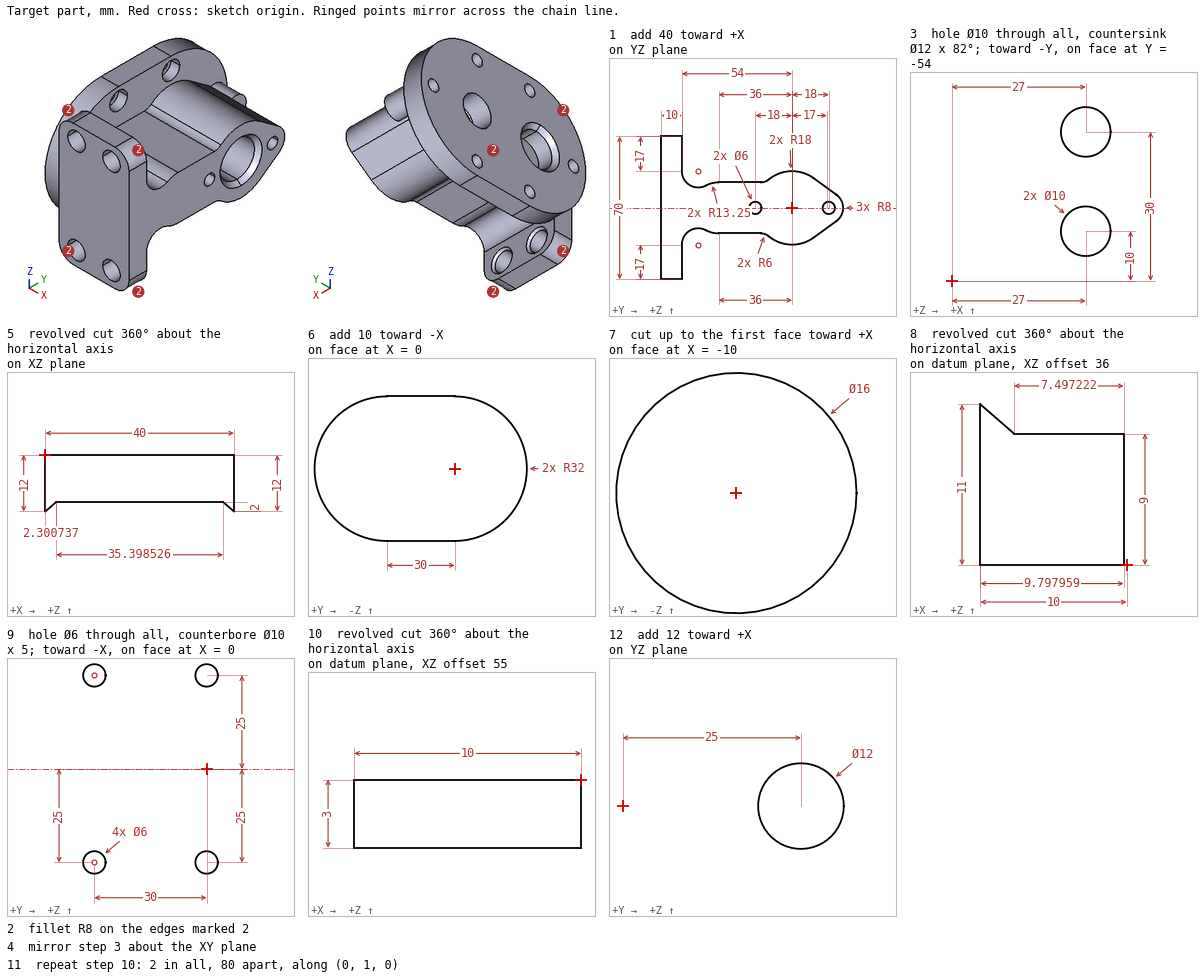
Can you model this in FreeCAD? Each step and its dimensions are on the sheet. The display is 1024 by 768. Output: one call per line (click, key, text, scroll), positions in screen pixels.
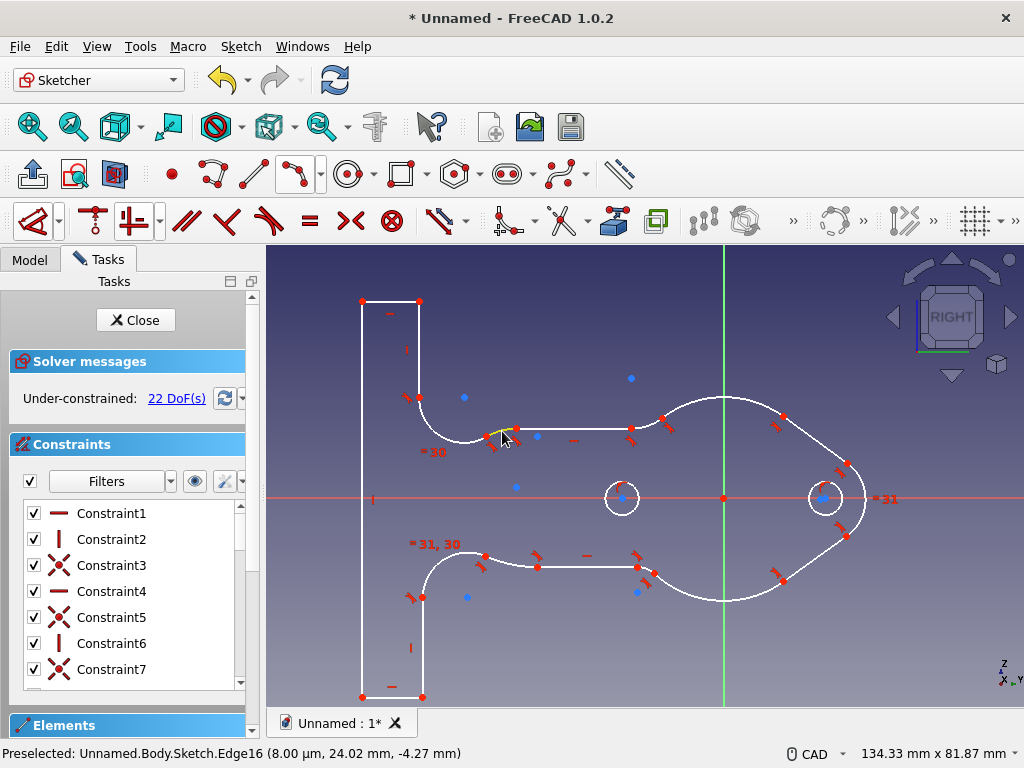
click(501, 431)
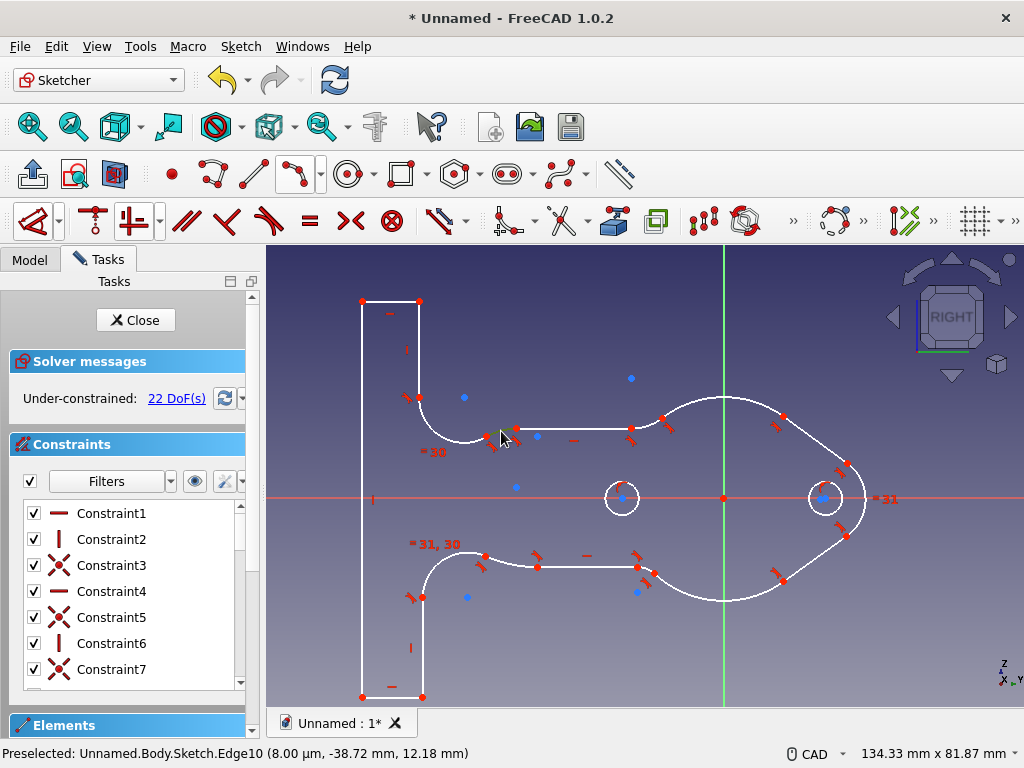
click(501, 562)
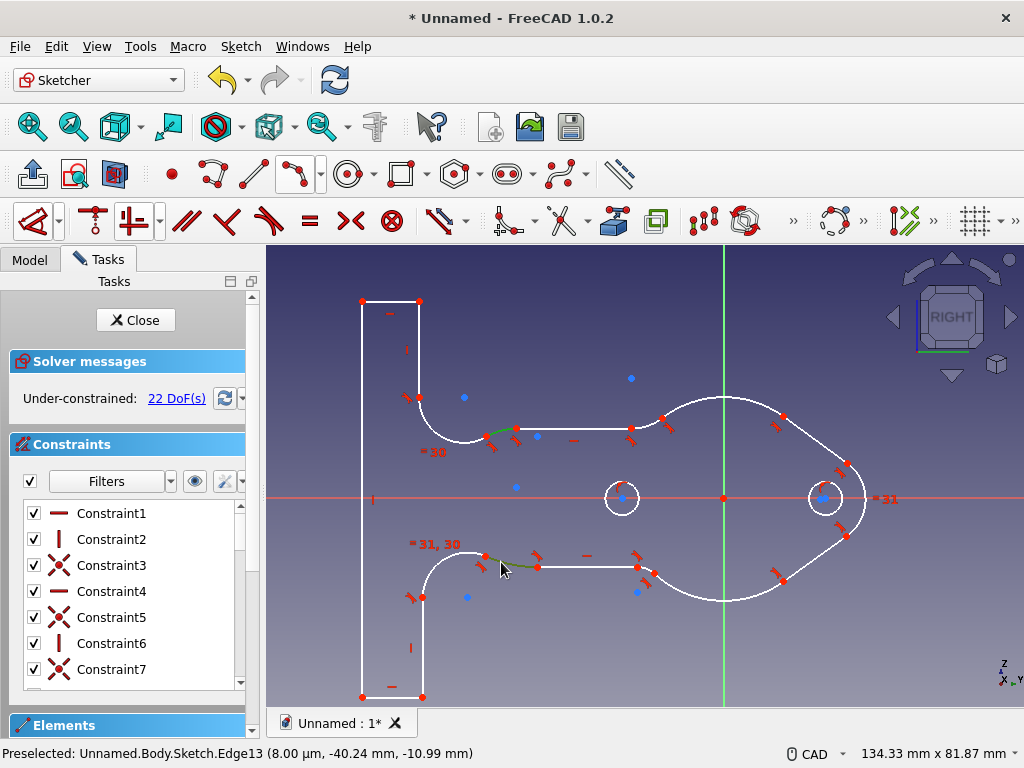
click(310, 222)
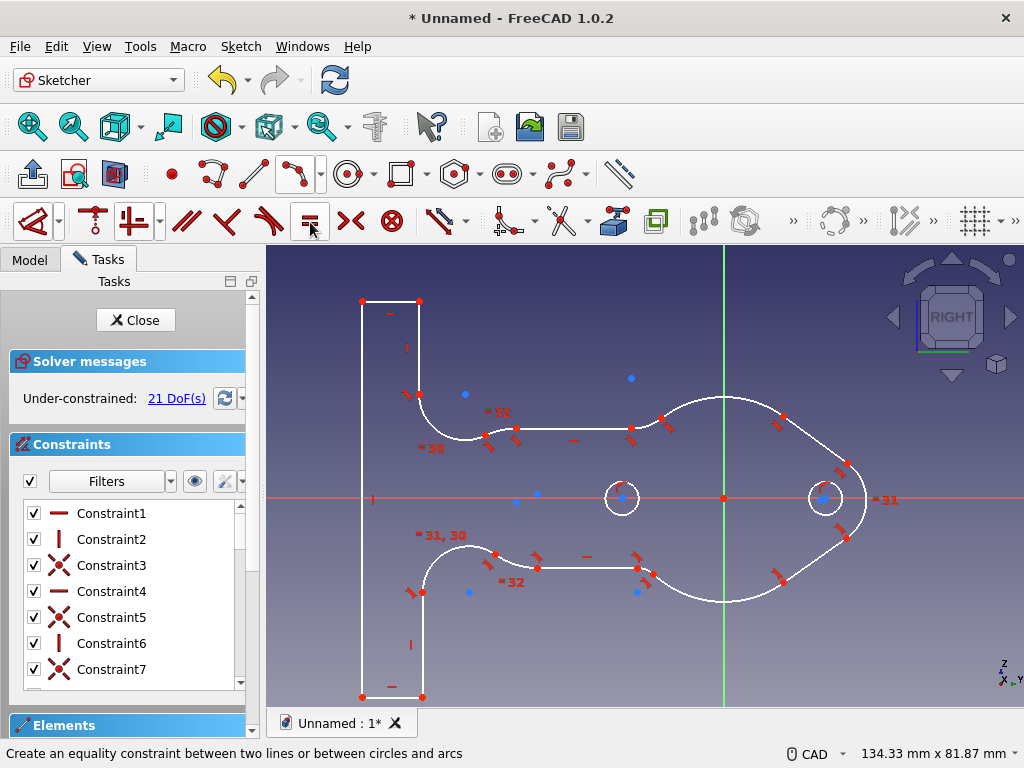
click(690, 596)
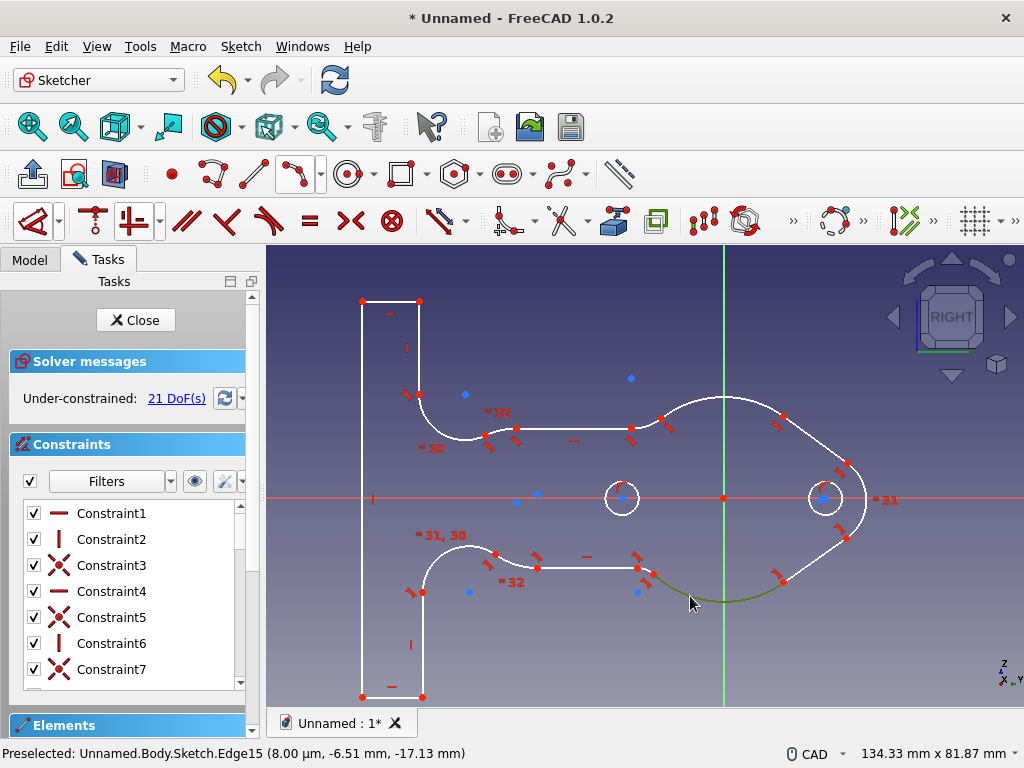
click(749, 400)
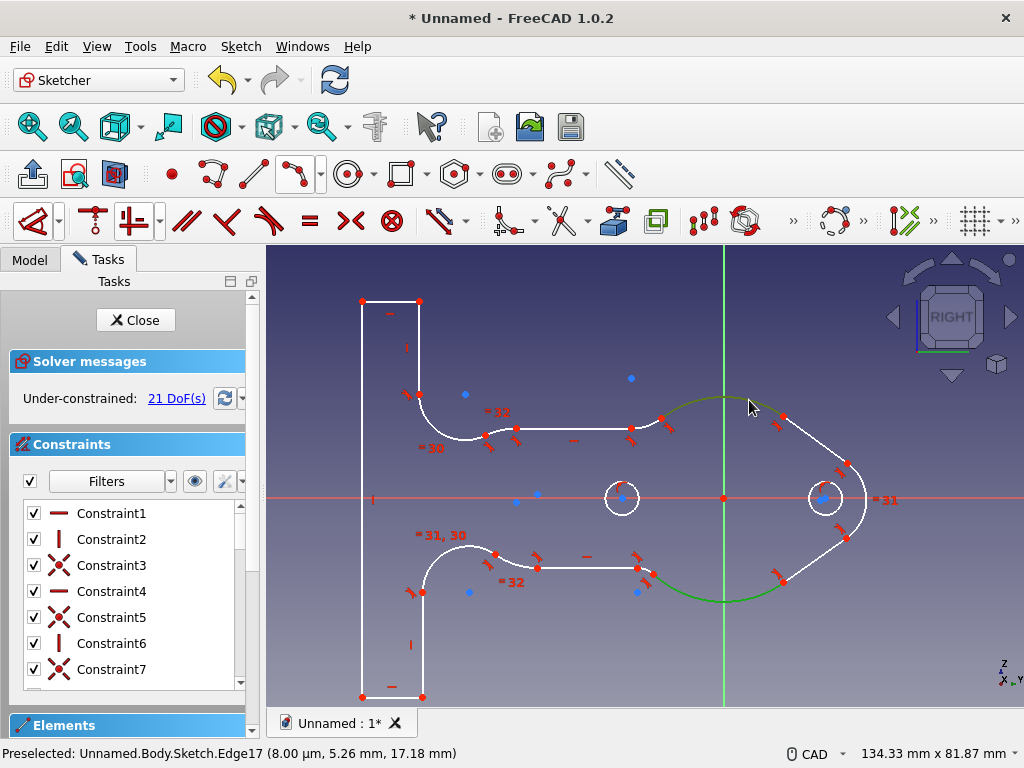
click(310, 222)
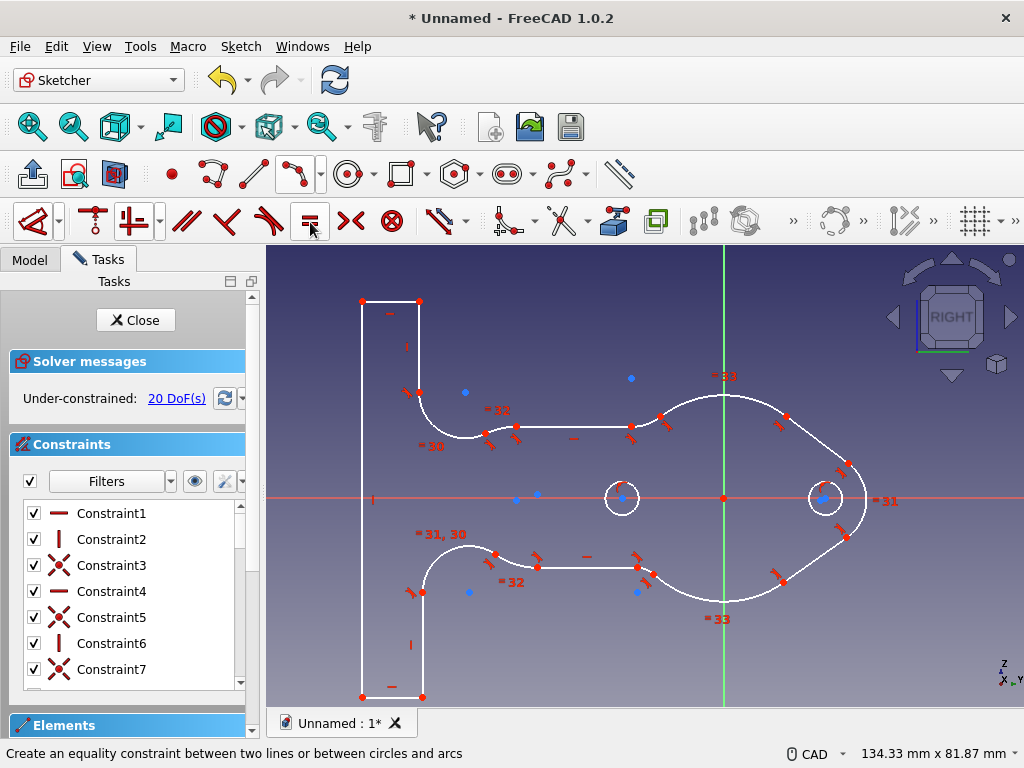
scroll(646, 570, up, 3)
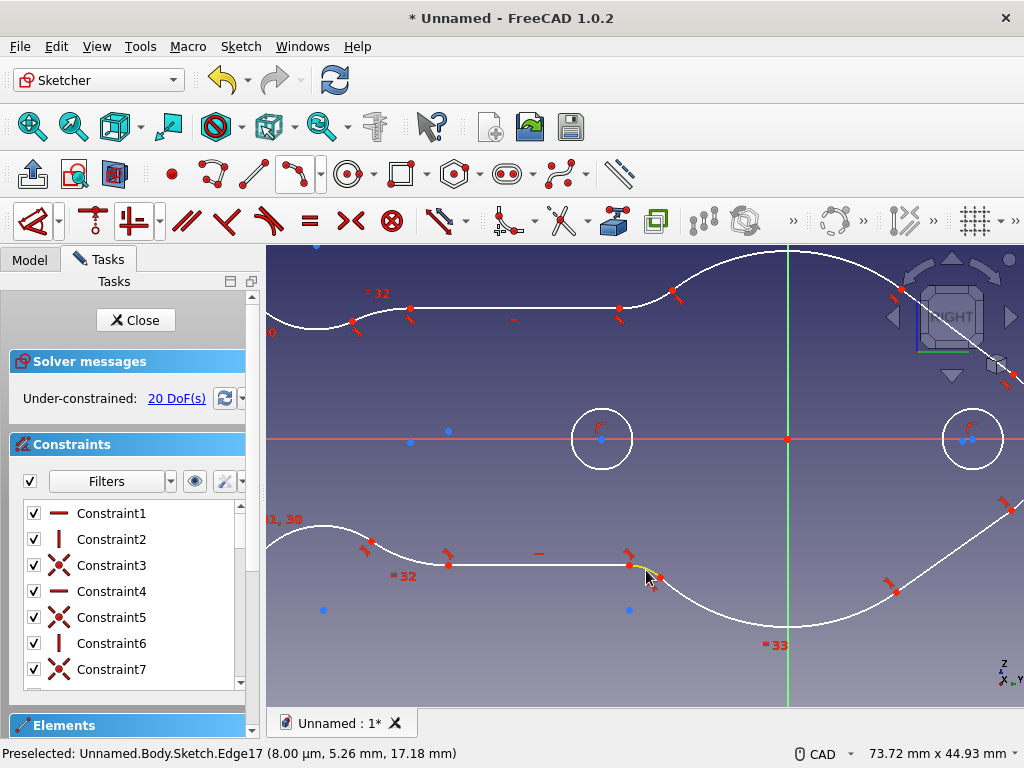
click(646, 569)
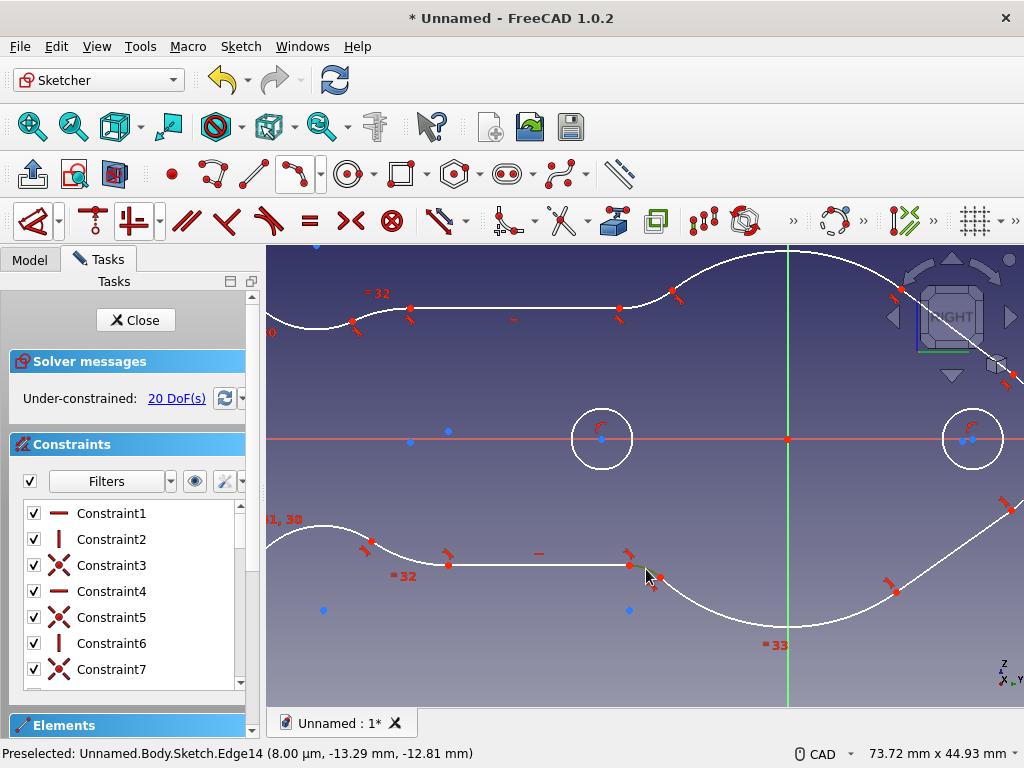
click(636, 307)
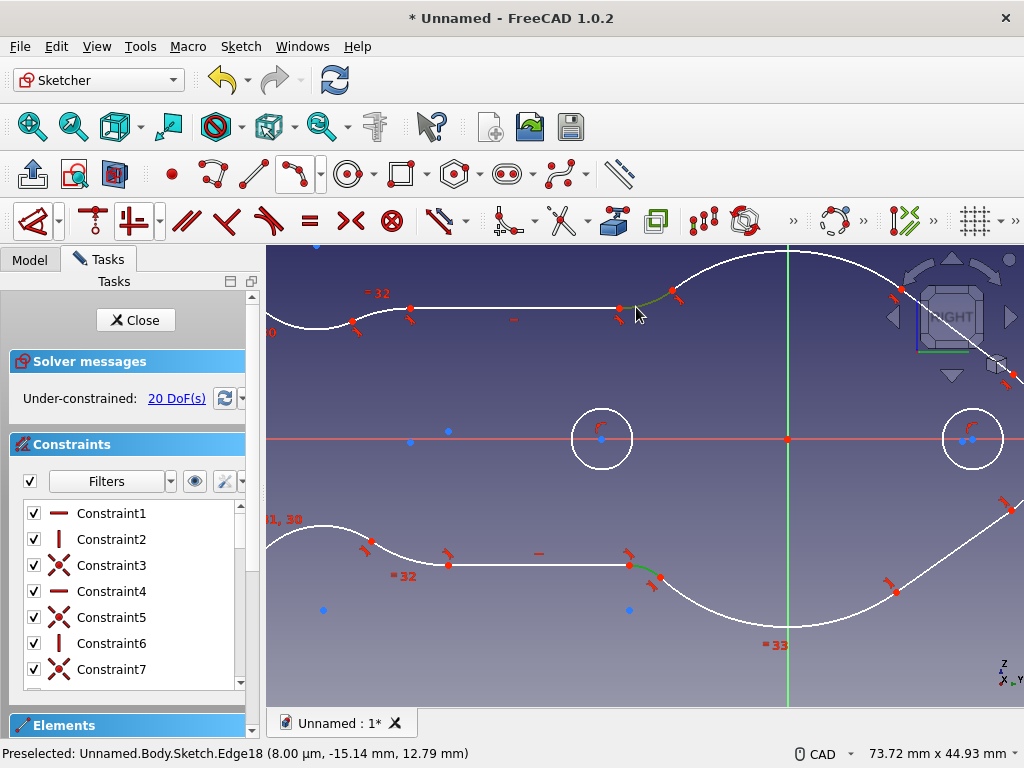
click(310, 222)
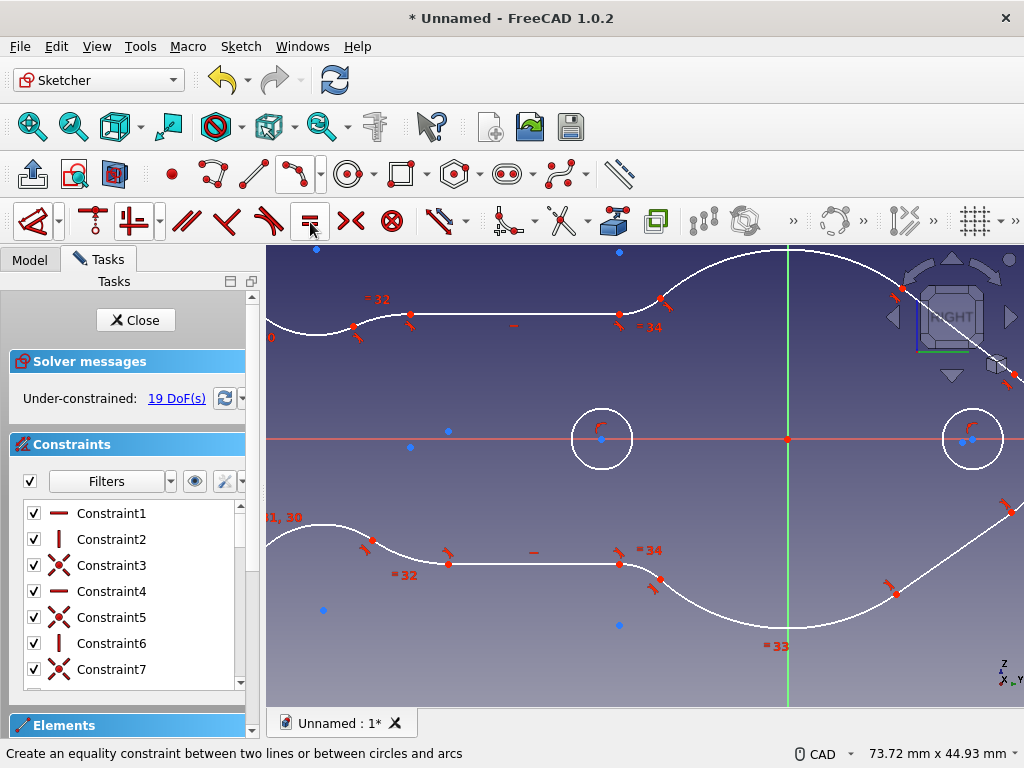
click(623, 418)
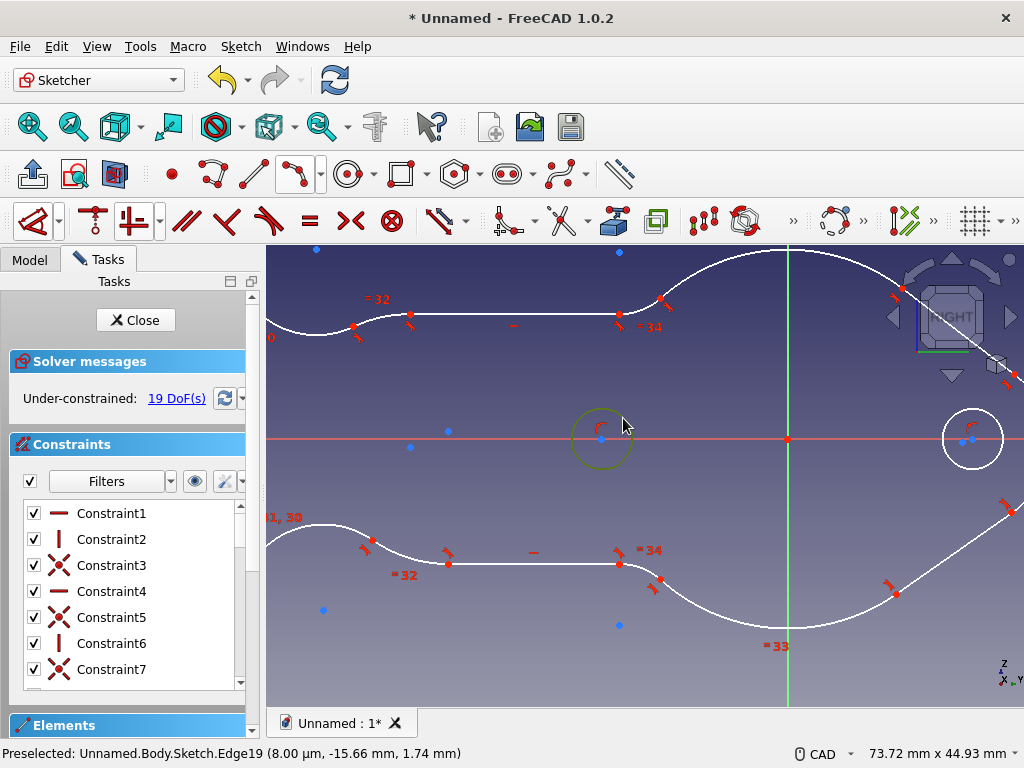
scroll(570, 497, down, 5)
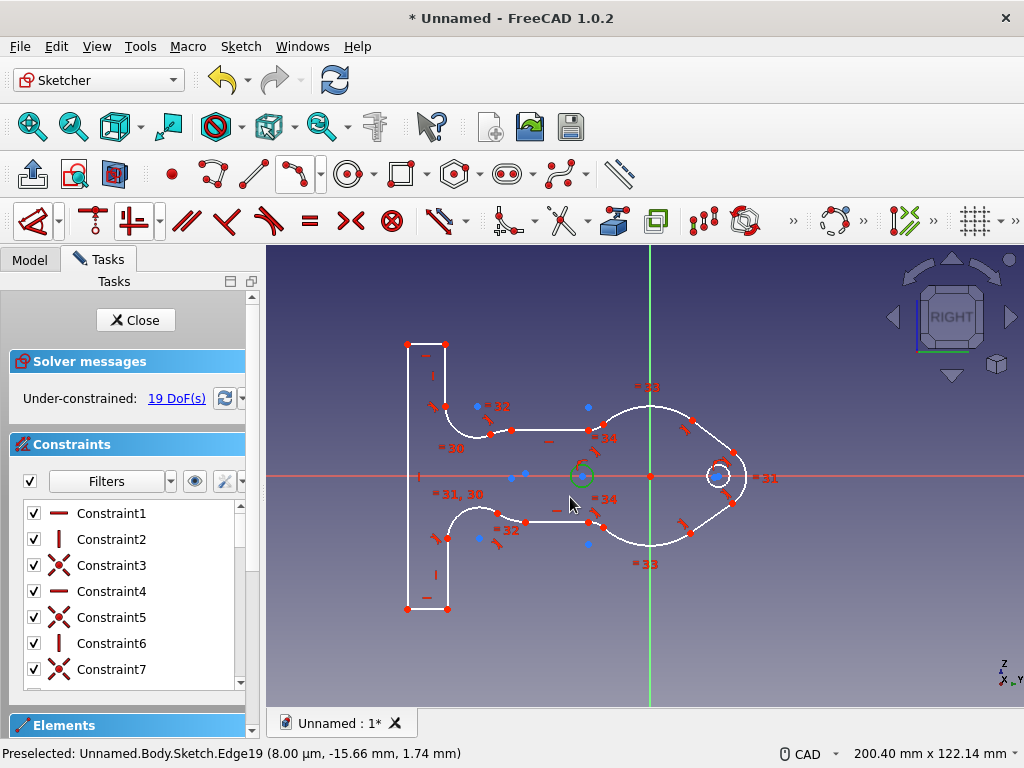
scroll(726, 468, up, 3)